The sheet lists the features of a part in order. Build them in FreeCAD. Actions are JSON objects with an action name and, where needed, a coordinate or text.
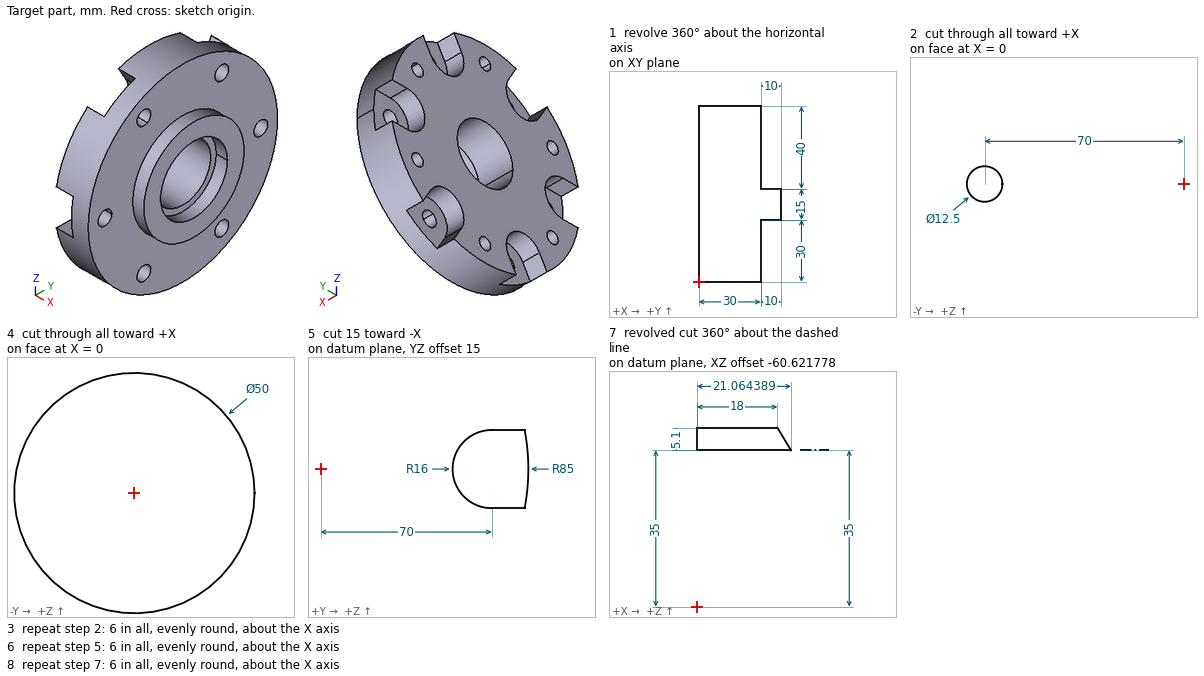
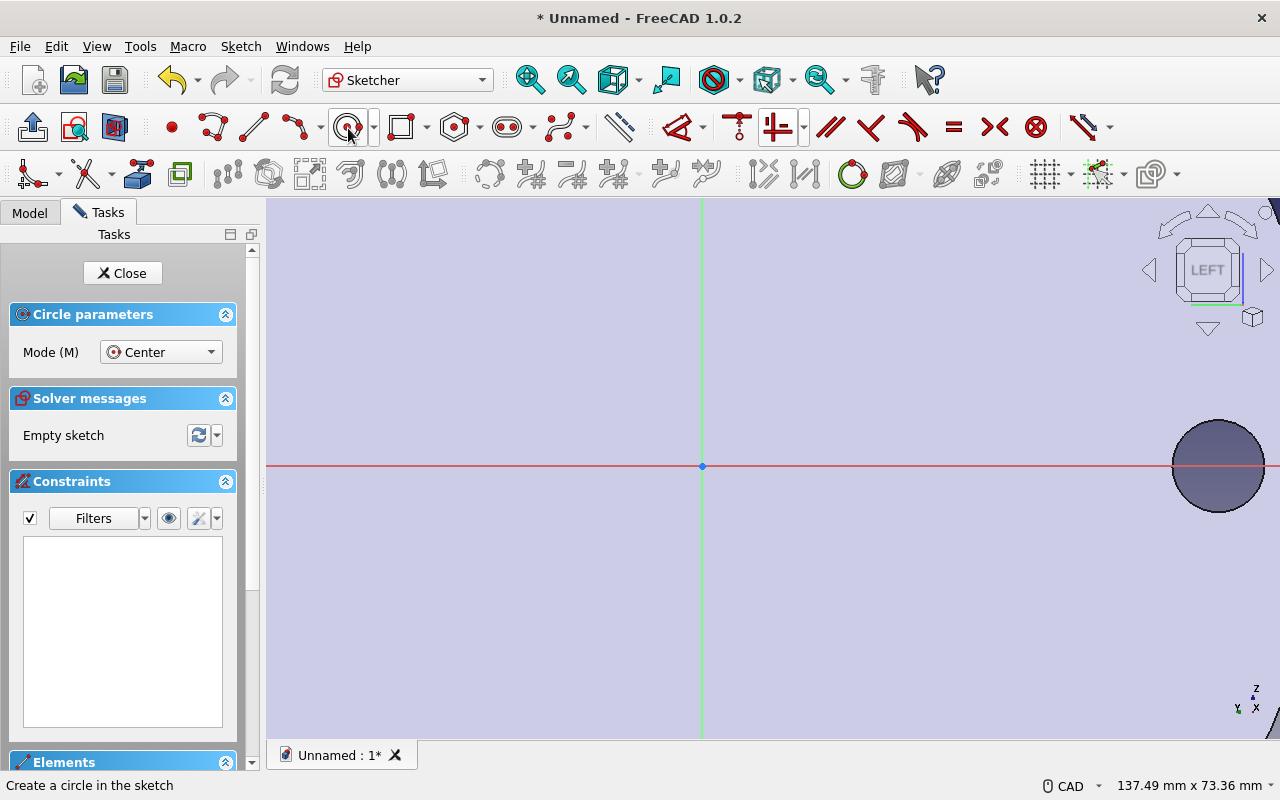
{"action": "left_click", "coordinate": [702, 466]}
{"action": "left_click", "coordinate": [833, 336]}
{"action": "key", "text": "Escape"}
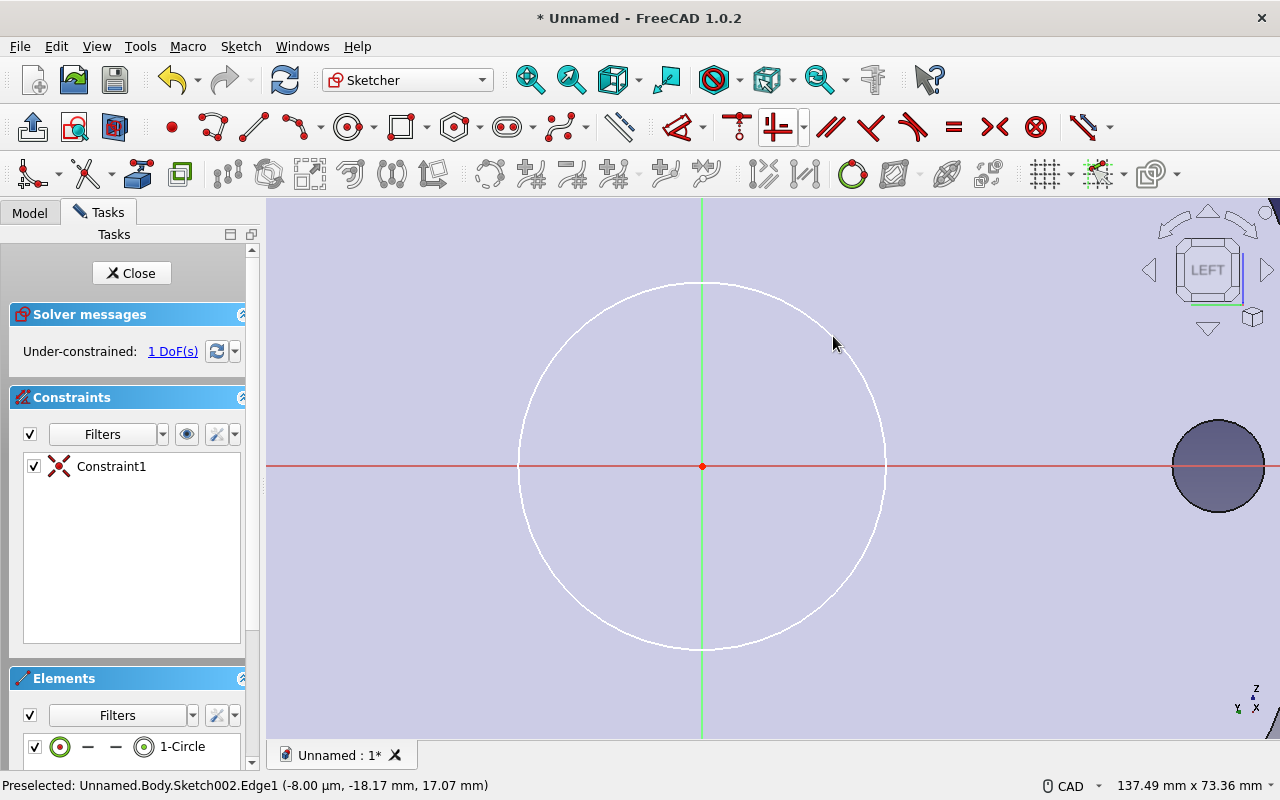
{"action": "left_click", "coordinate": [676, 128]}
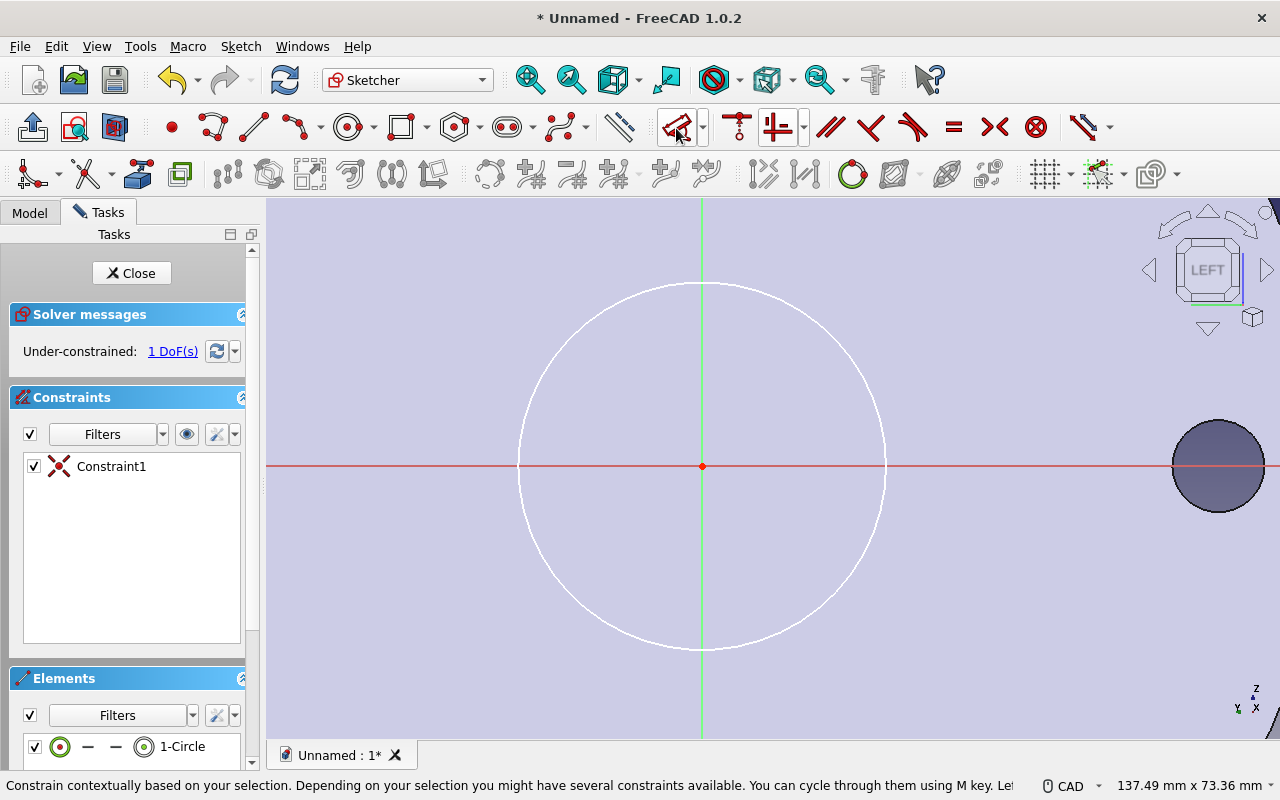
{"action": "left_click", "coordinate": [832, 336]}
{"action": "left_click", "coordinate": [855, 313]}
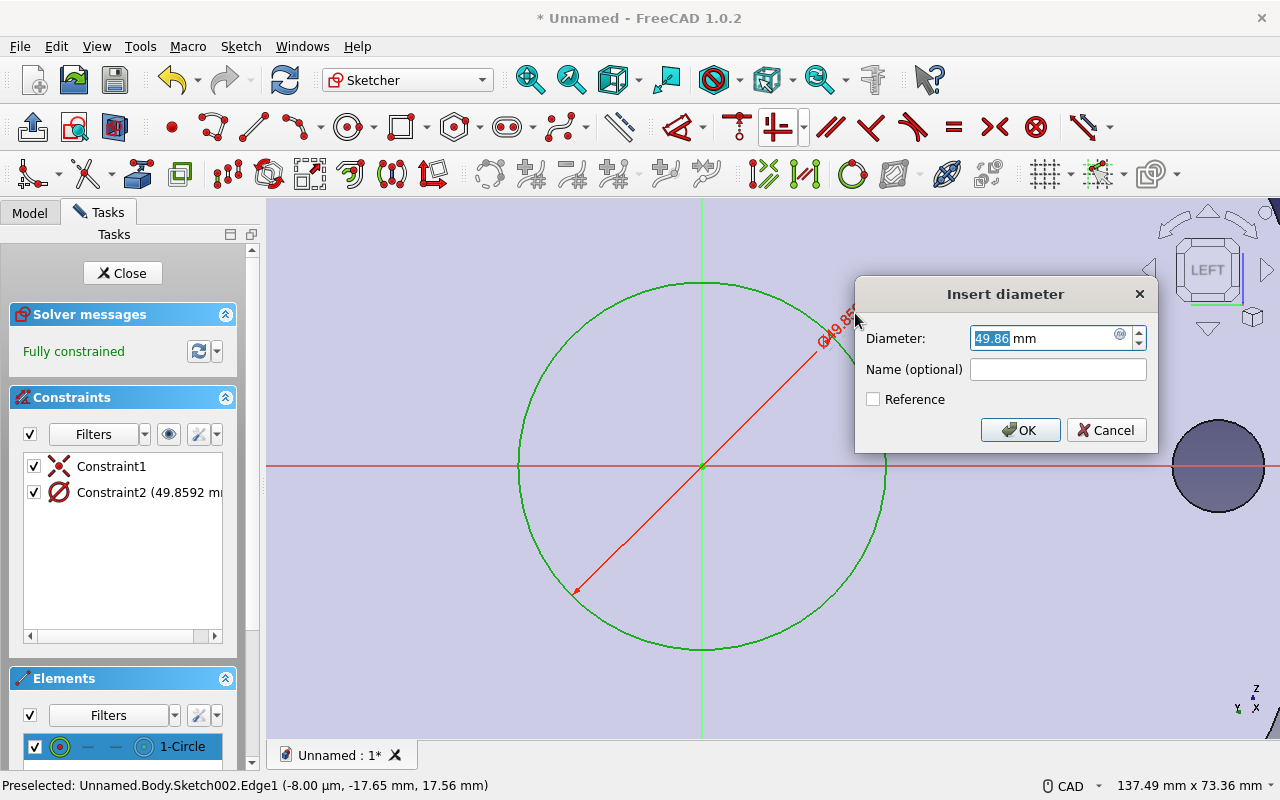
{"action": "type", "text": "50"}
{"action": "key", "text": "Return"}
{"action": "key", "text": "Escape"}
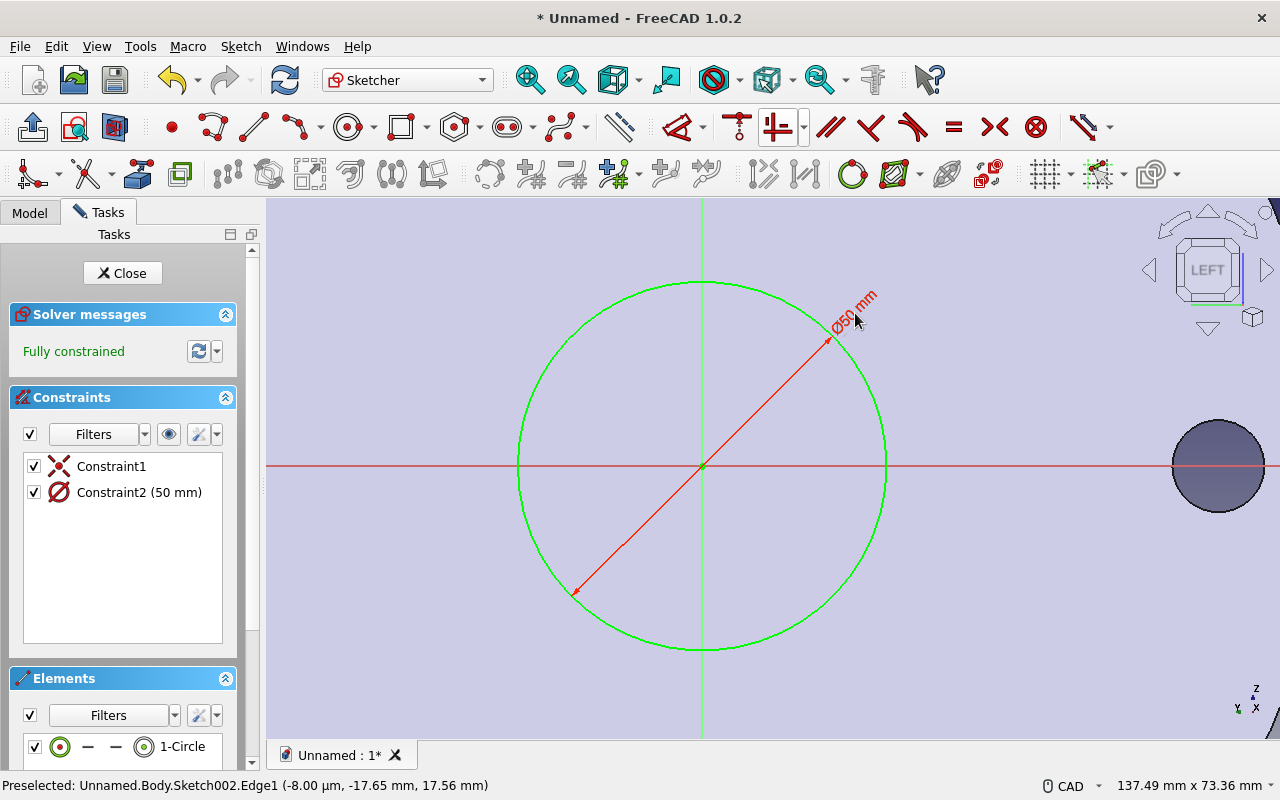
{"action": "left_click", "coordinate": [123, 273]}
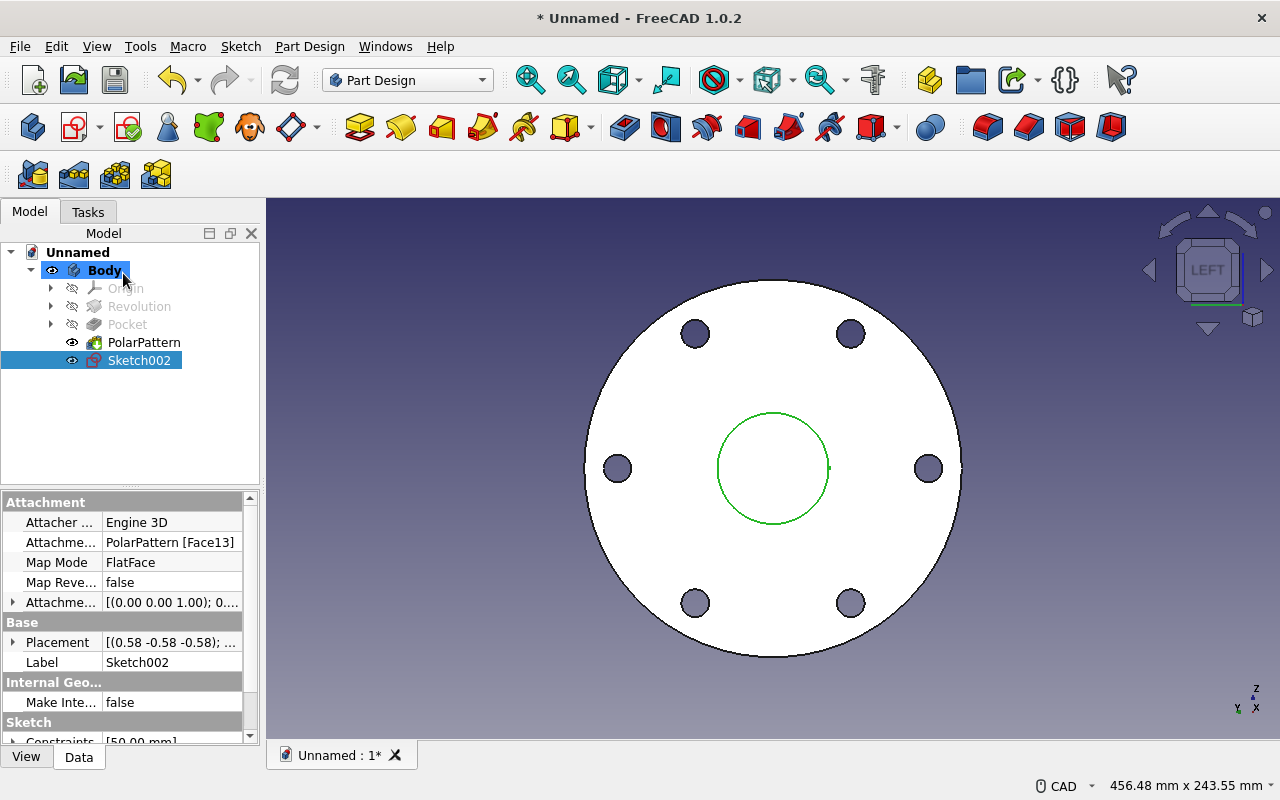
{"action": "left_click", "coordinate": [625, 128]}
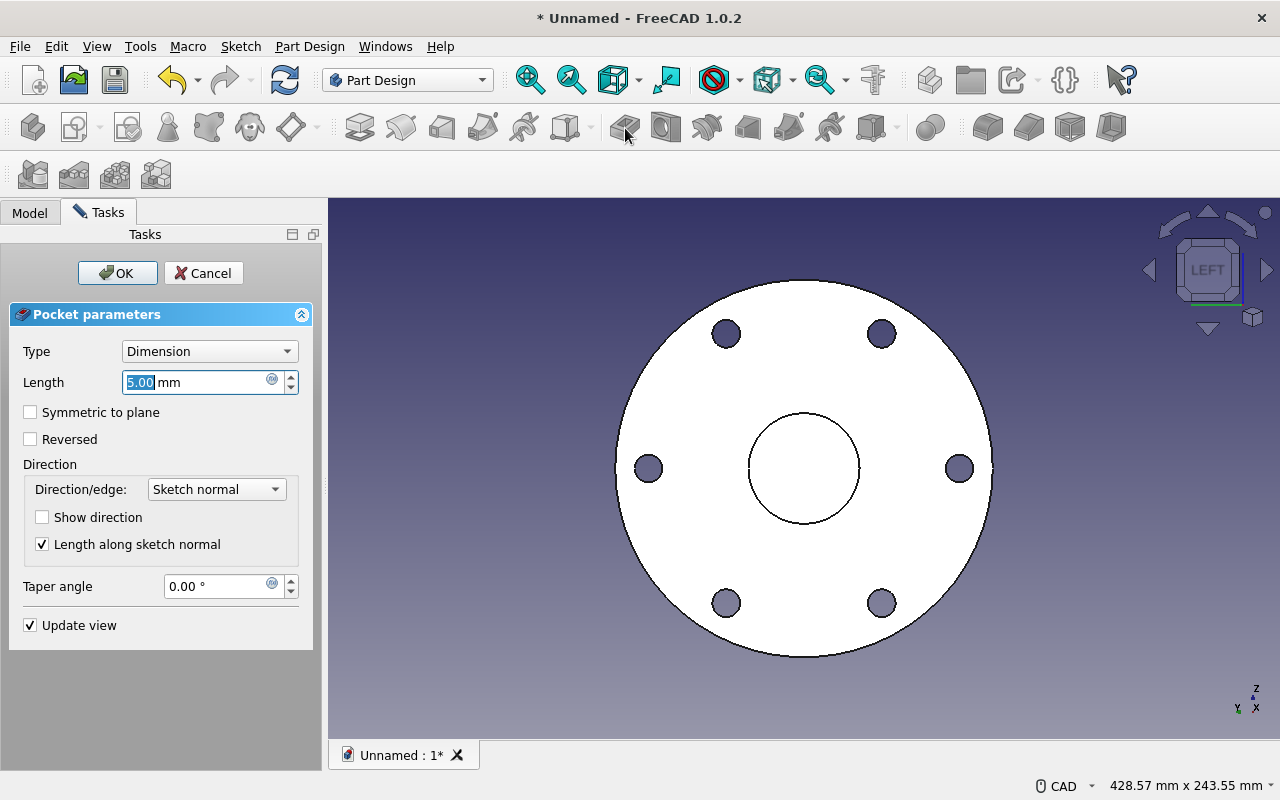
{"action": "left_click", "coordinate": [210, 352]}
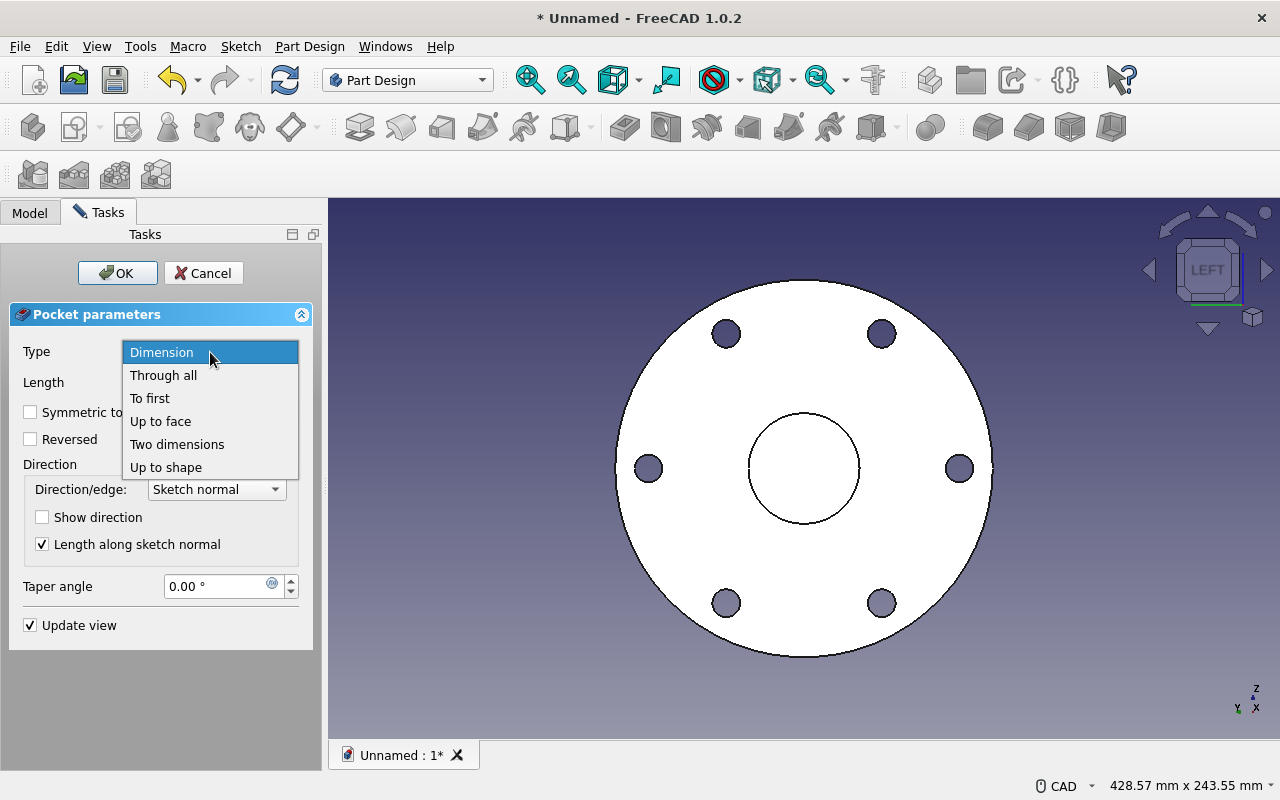
{"action": "left_click", "coordinate": [208, 376]}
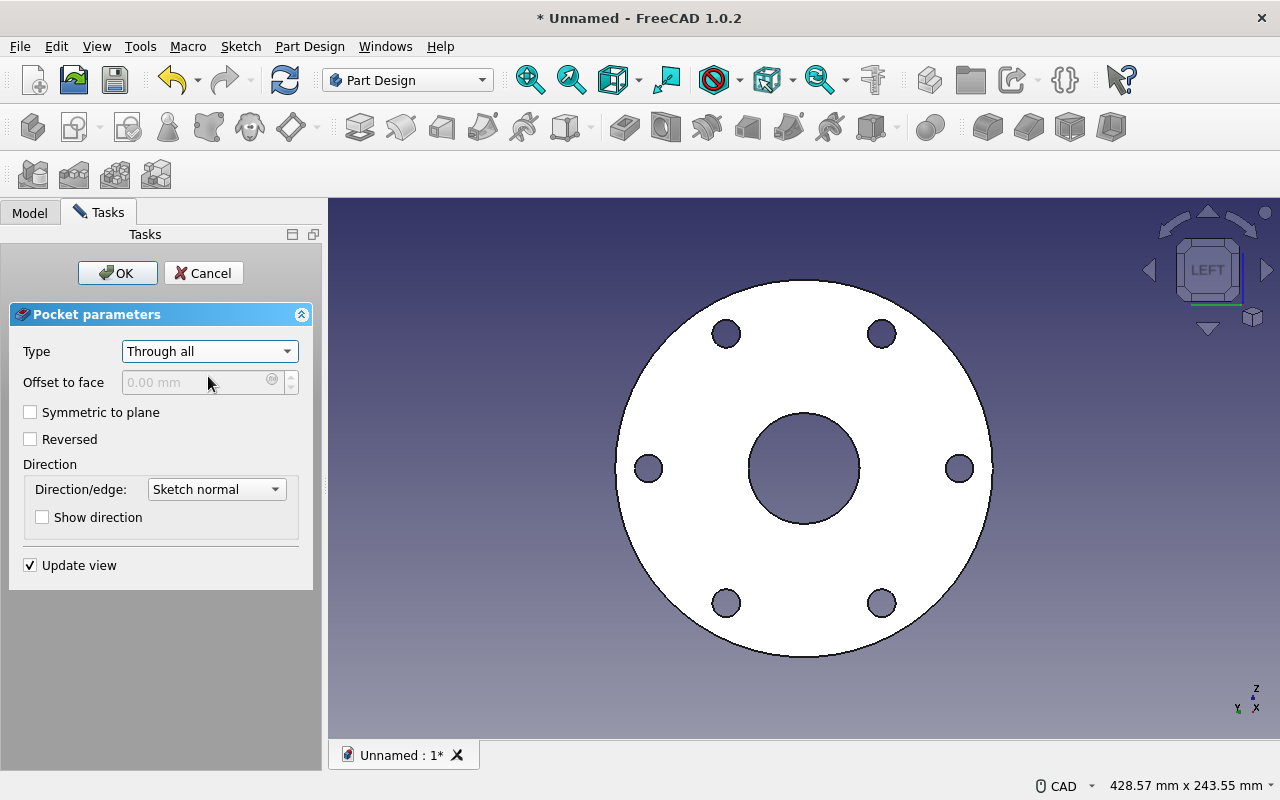
{"action": "left_click", "coordinate": [118, 273]}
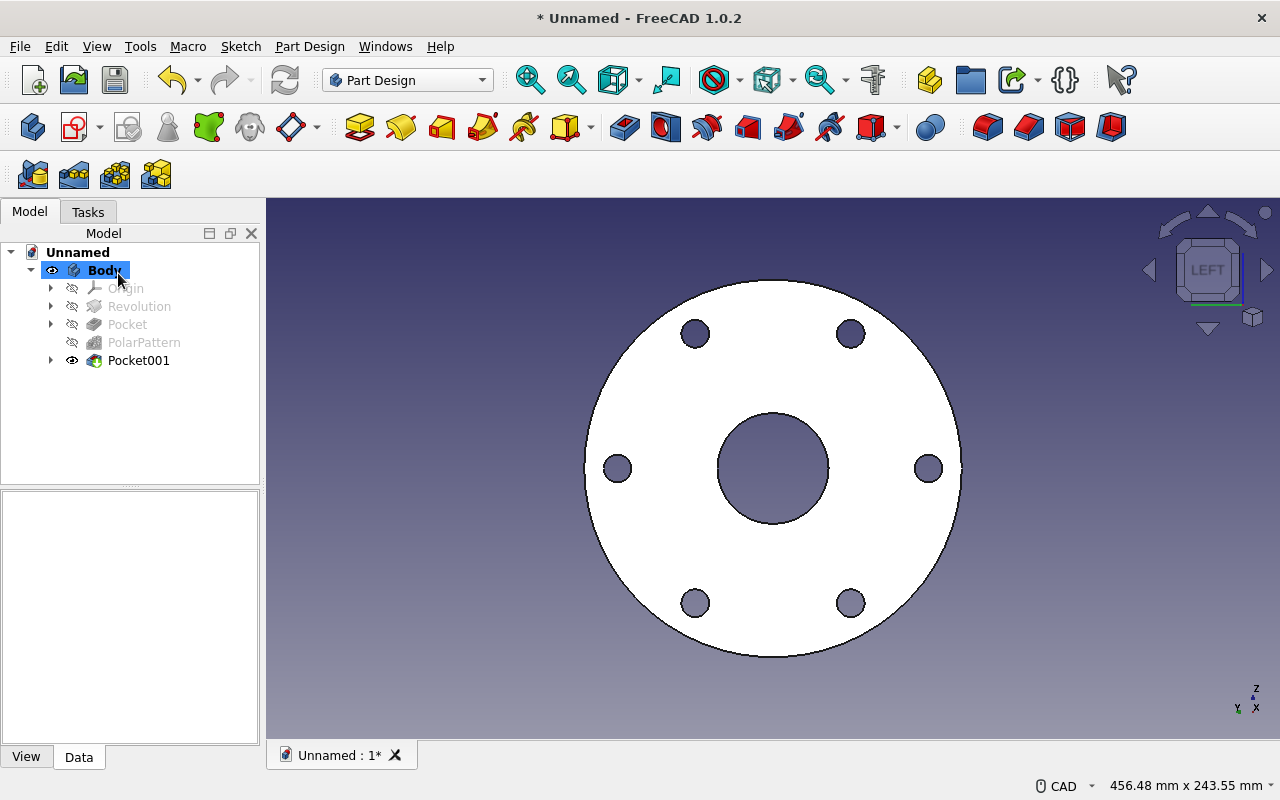
{"action": "left_click", "coordinate": [51, 288]}